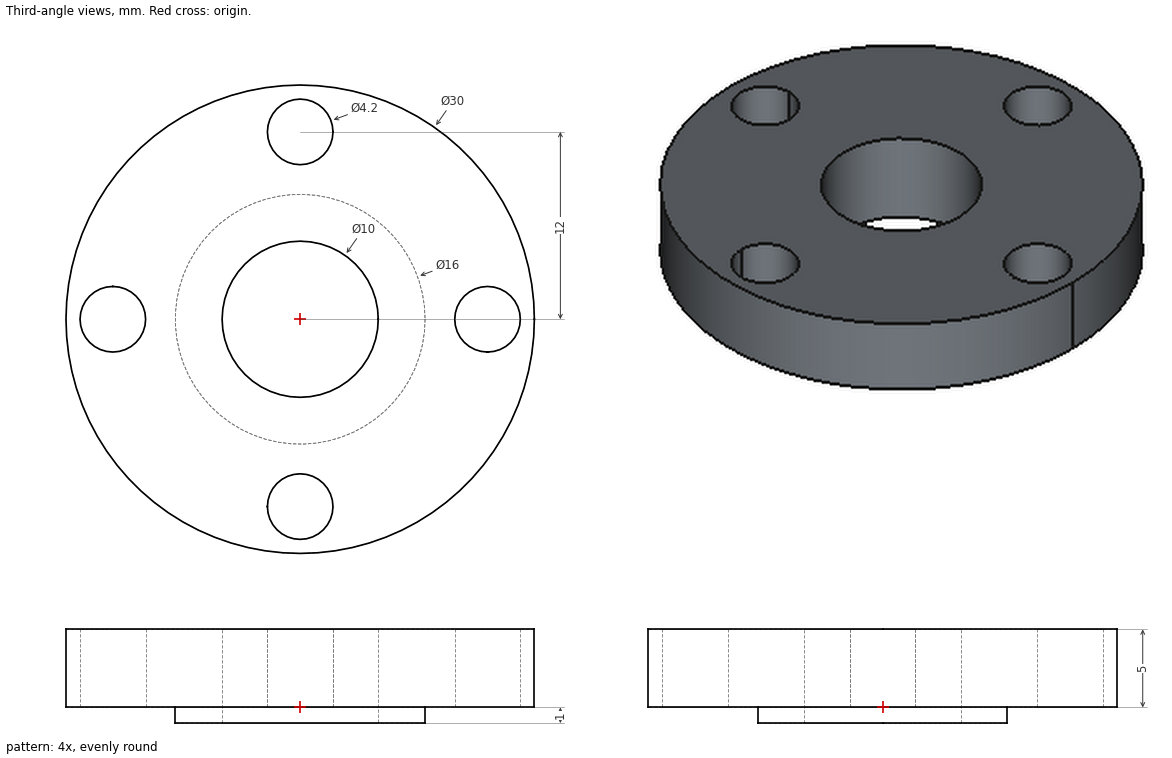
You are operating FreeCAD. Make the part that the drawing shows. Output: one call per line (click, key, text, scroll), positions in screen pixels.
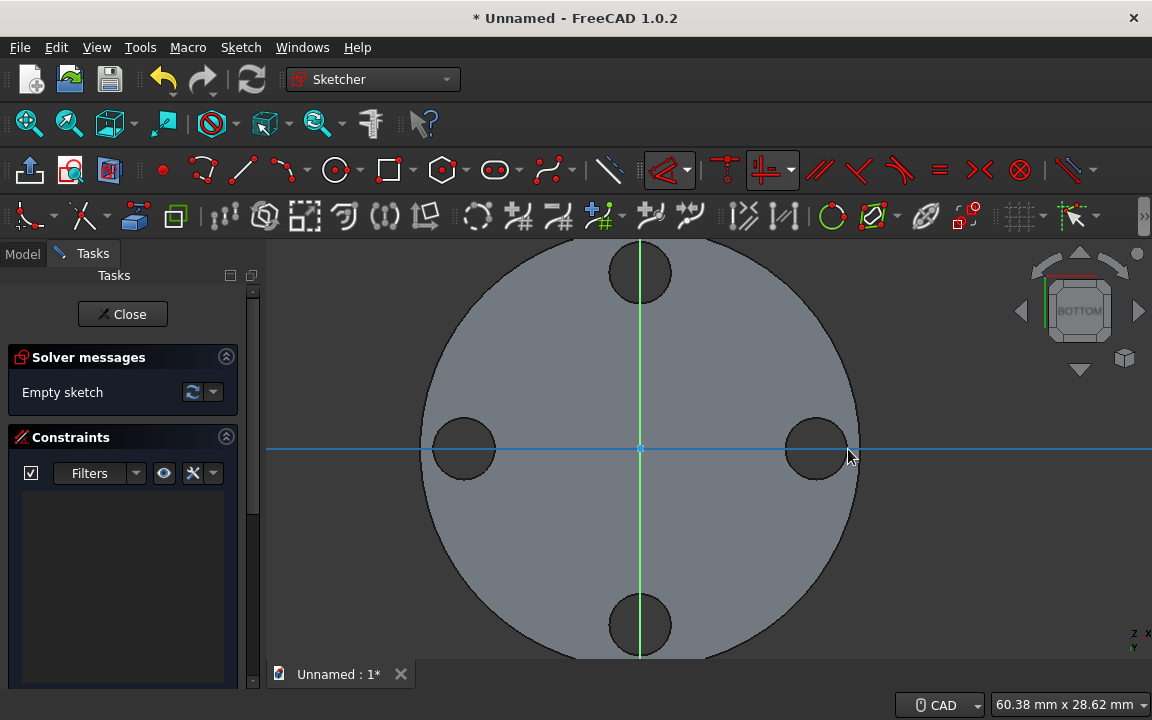
click(336, 170)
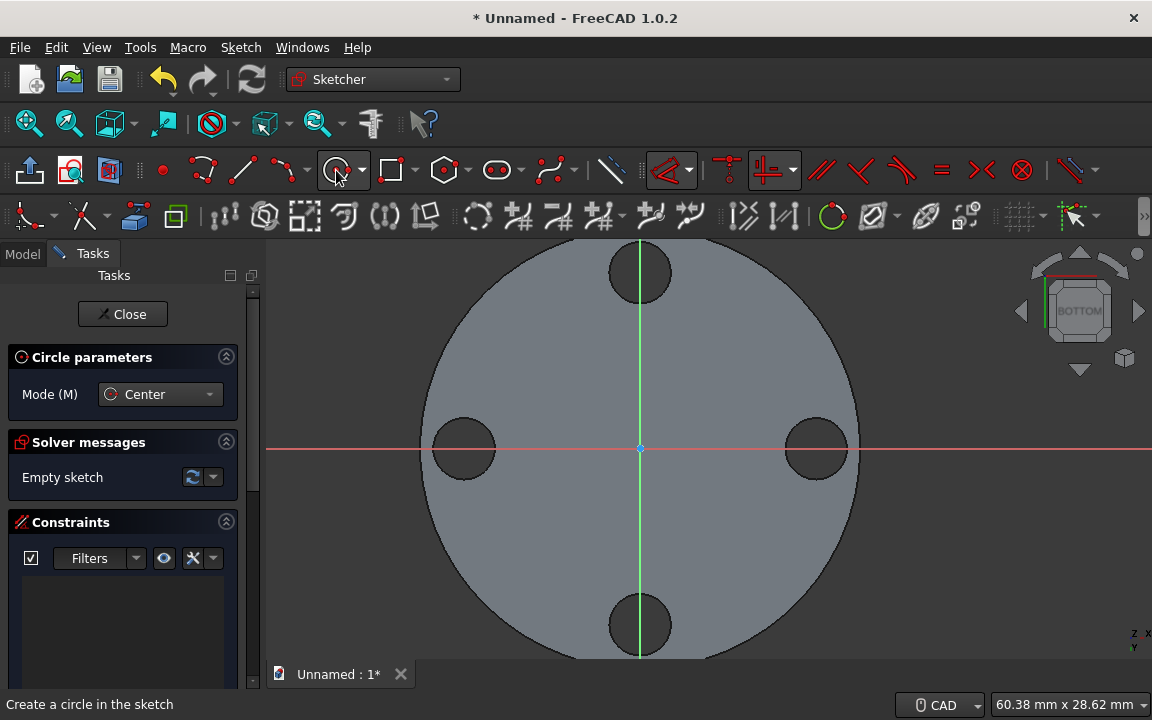
click(640, 449)
click(723, 366)
key(Escape)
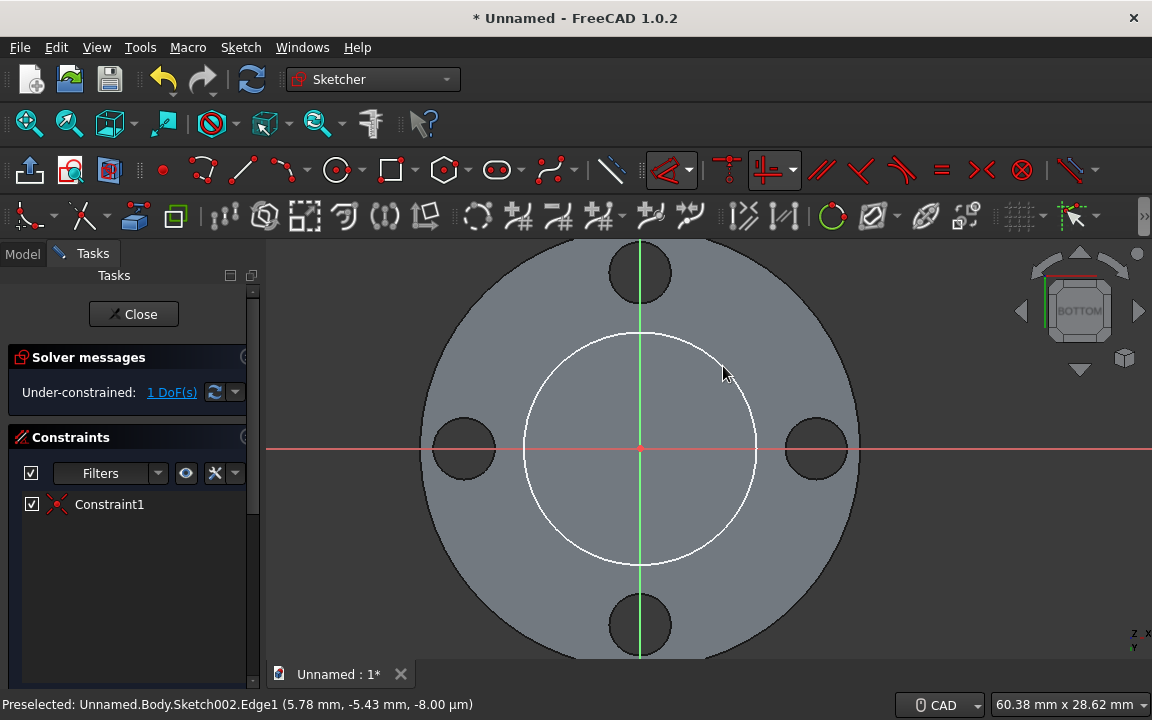
click(722, 366)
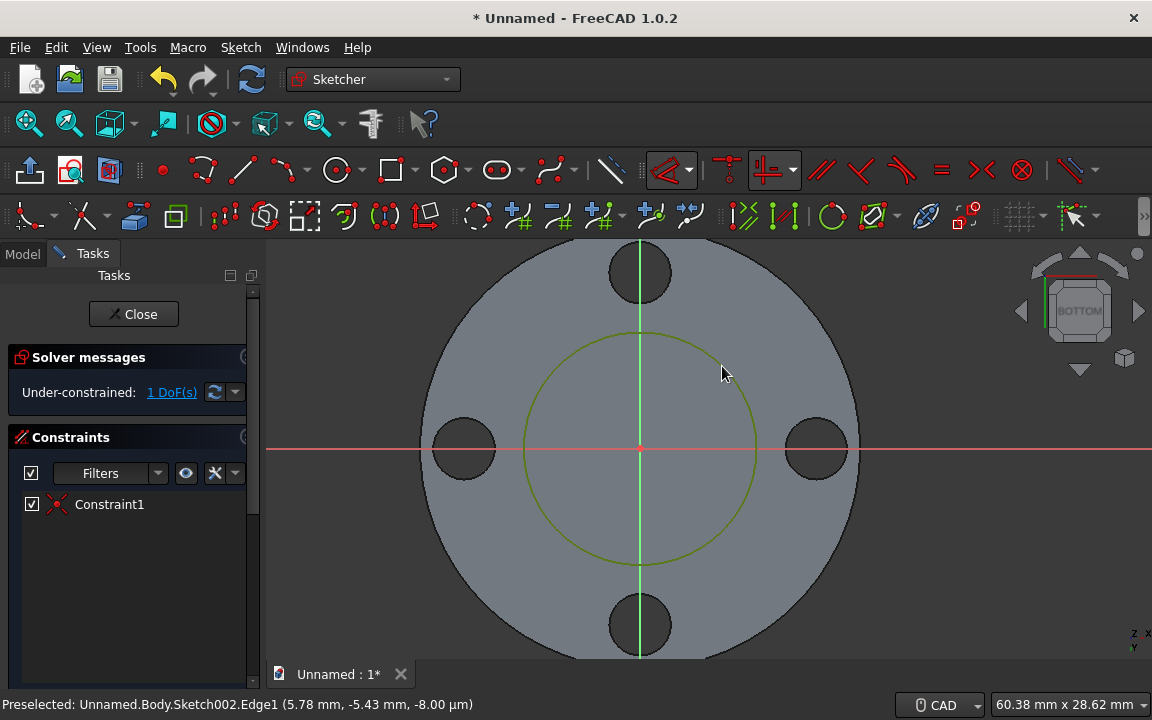
click(692, 170)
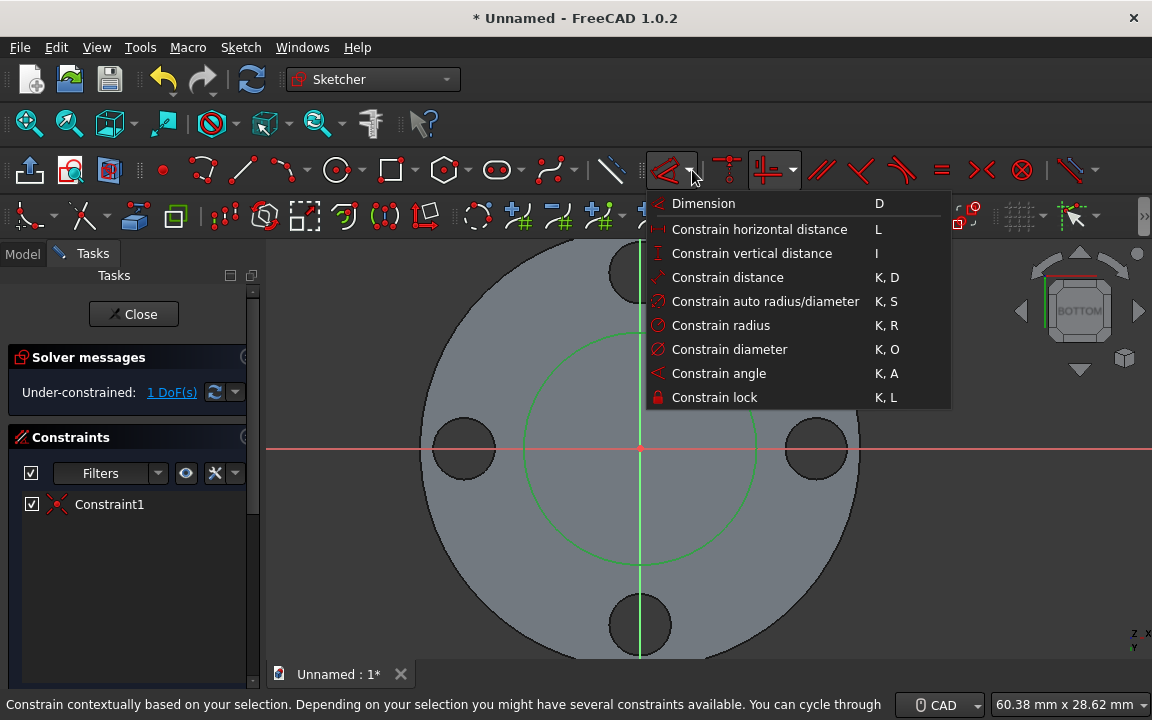
click(799, 349)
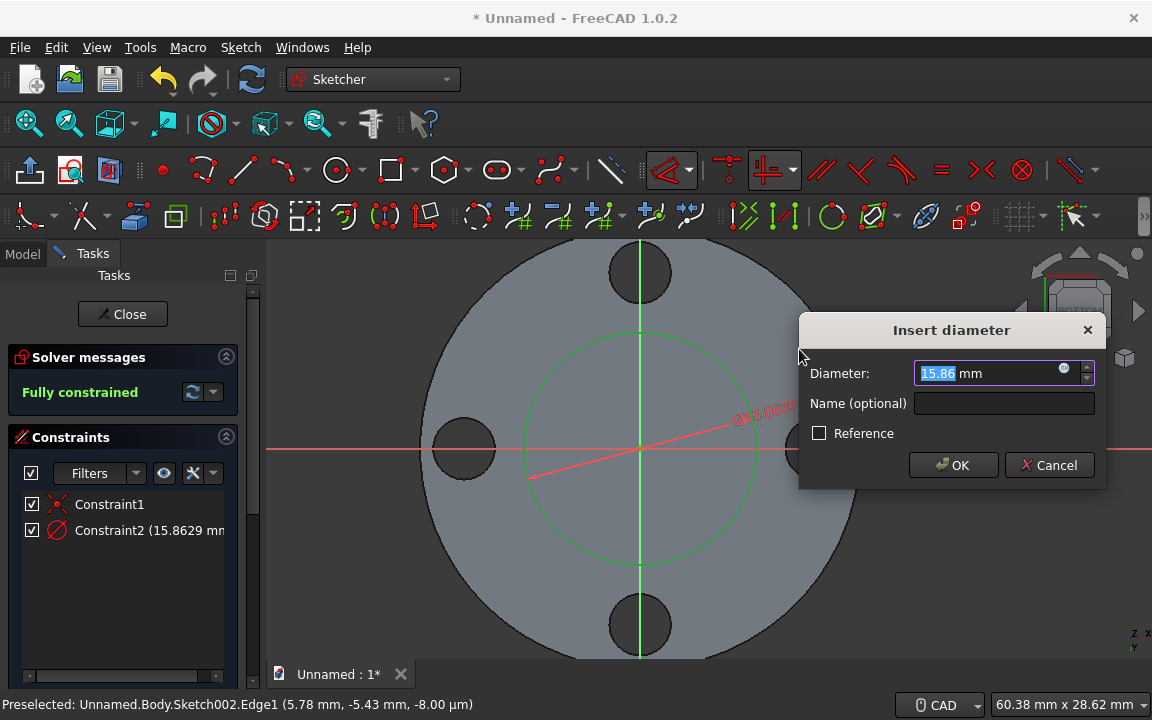
text(16)
key(Return)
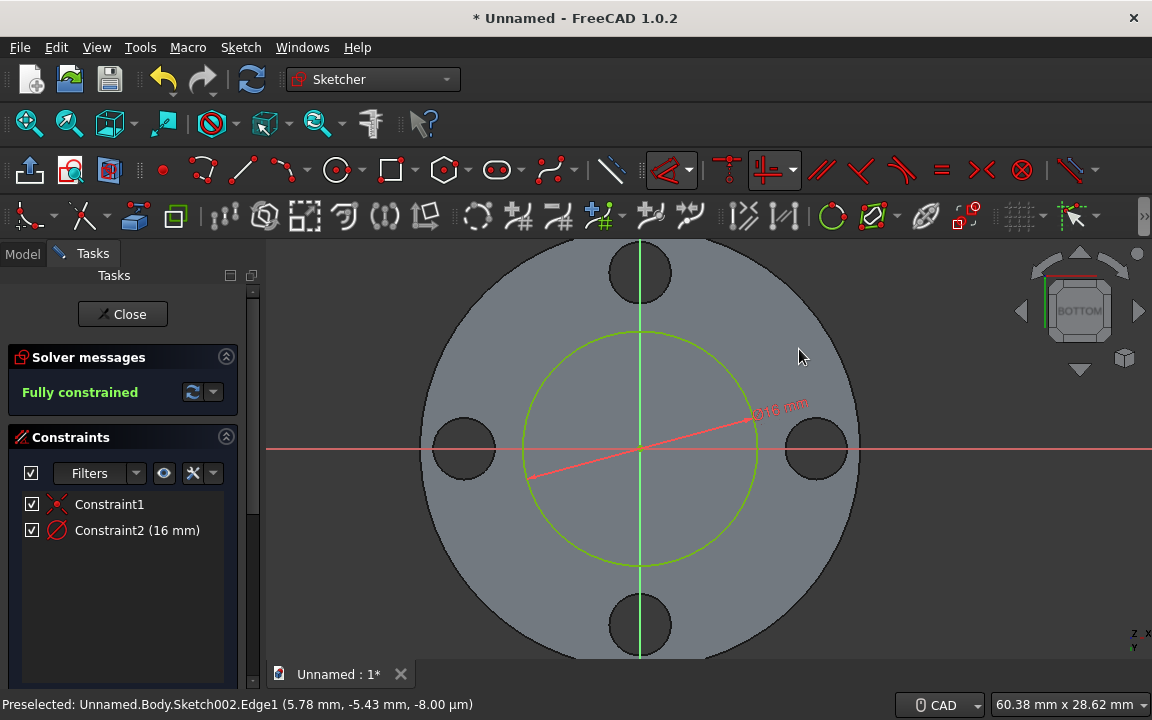
click(123, 314)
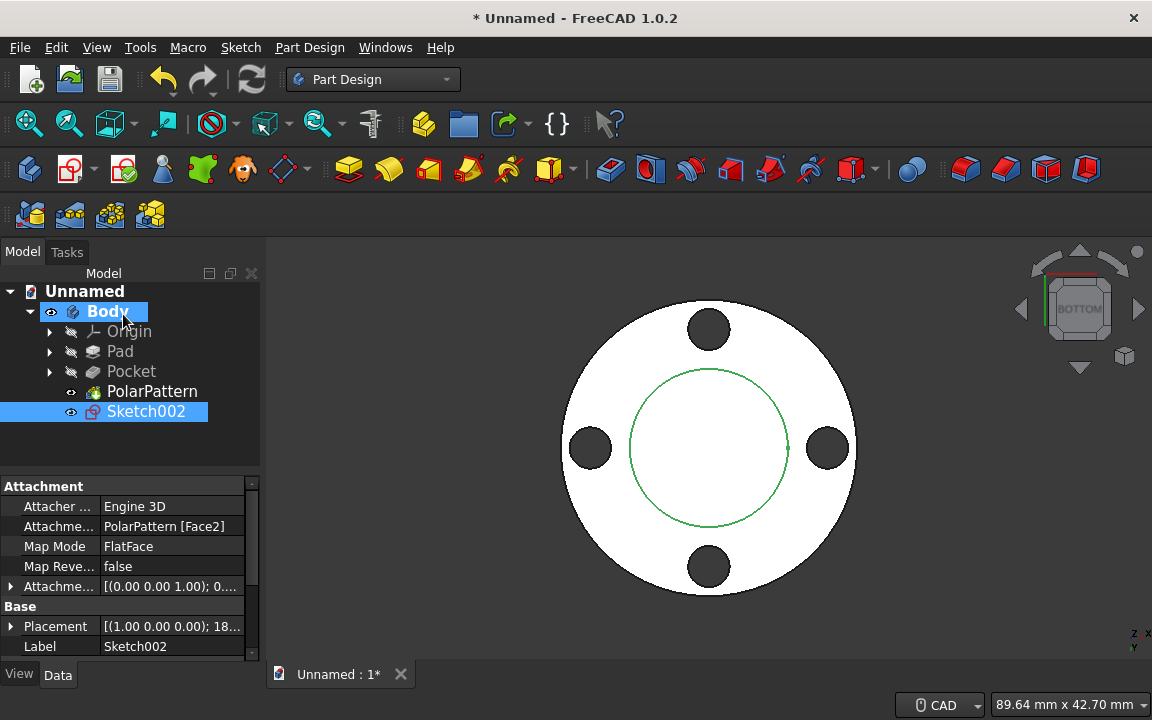
click(350, 170)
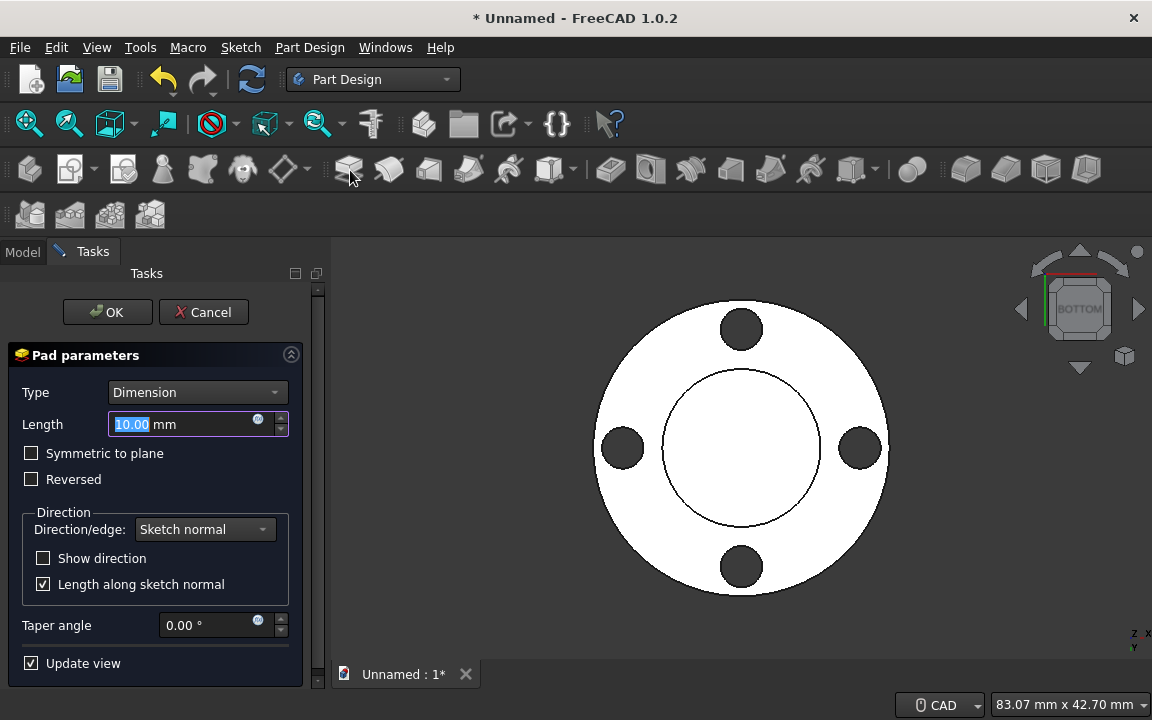
text(1)
key(Tab)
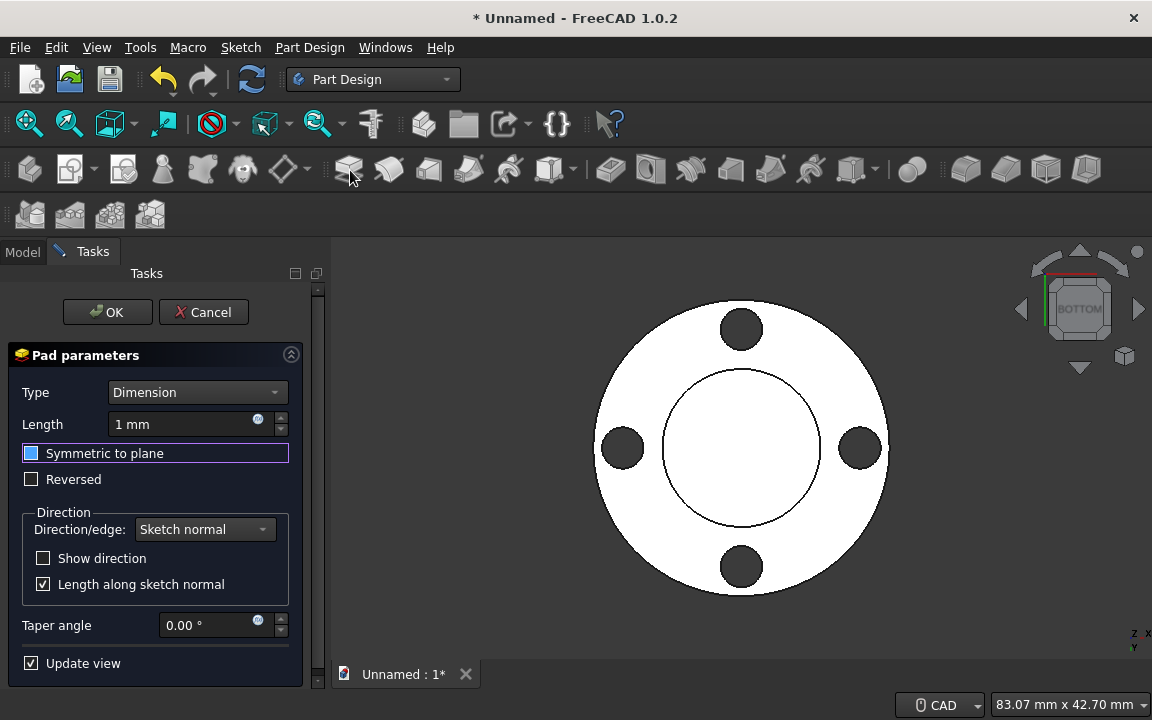
click(108, 312)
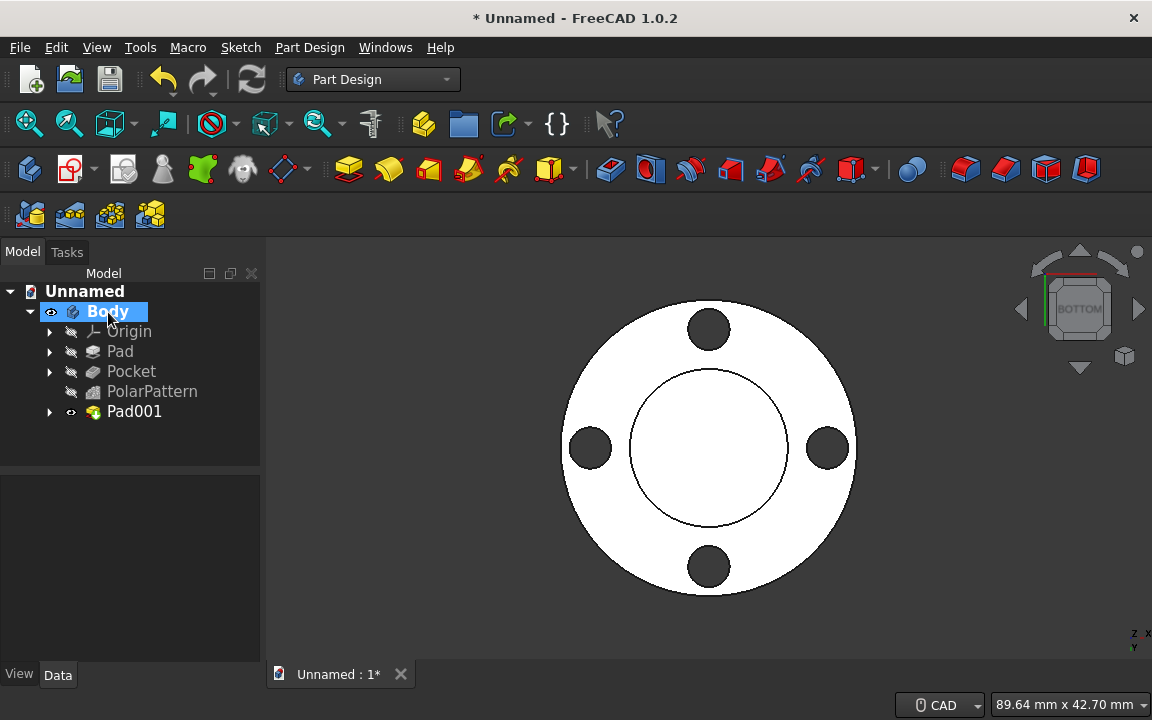
key(0)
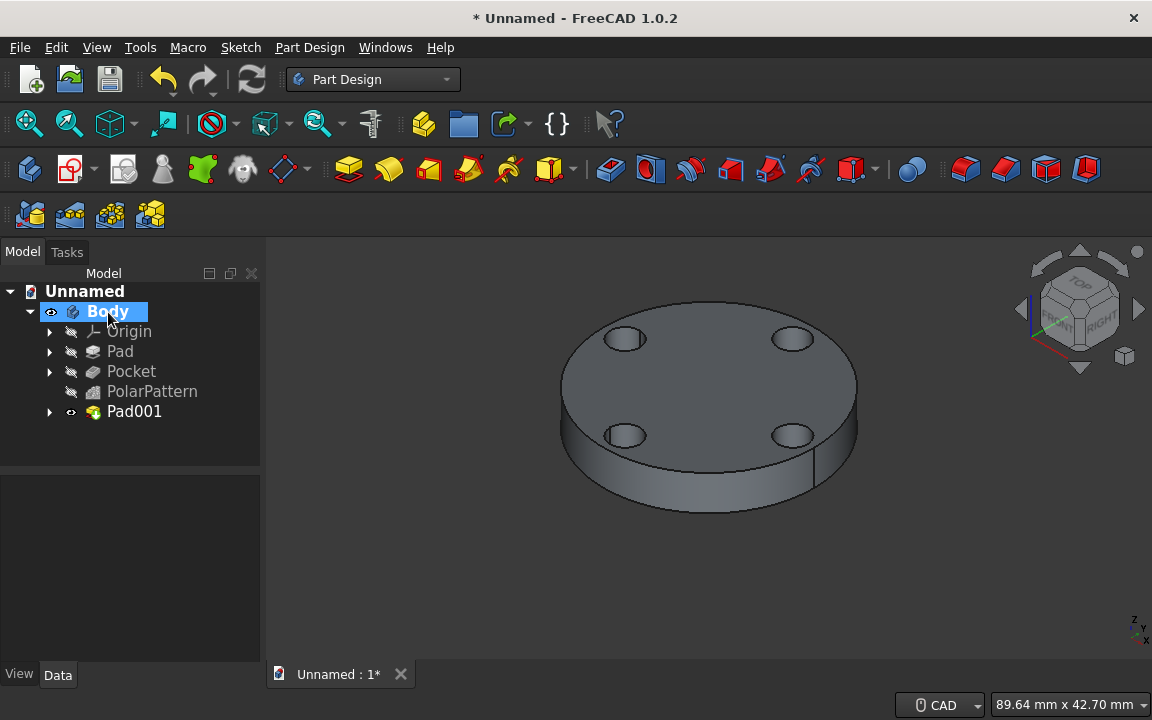
click(709, 386)